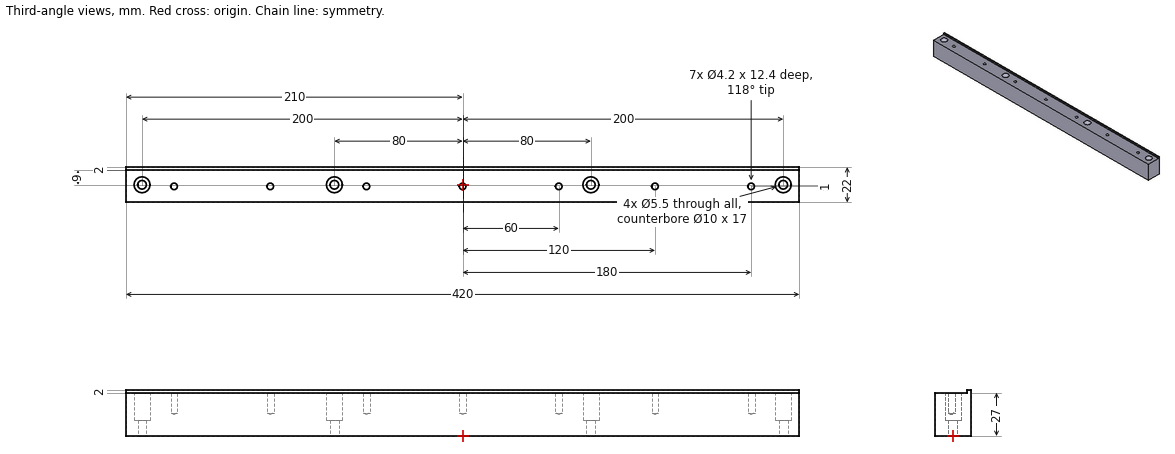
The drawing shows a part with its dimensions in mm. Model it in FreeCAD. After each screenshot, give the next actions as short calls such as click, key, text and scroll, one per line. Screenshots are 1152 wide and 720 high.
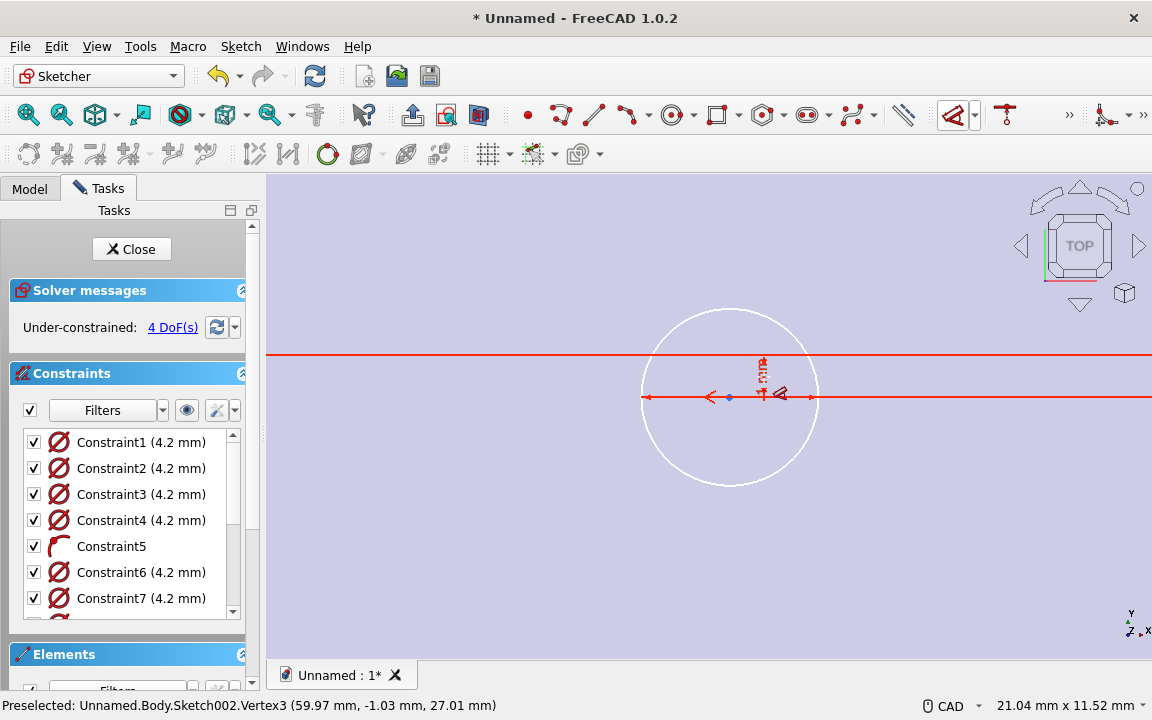
scroll(744, 417, down, 16)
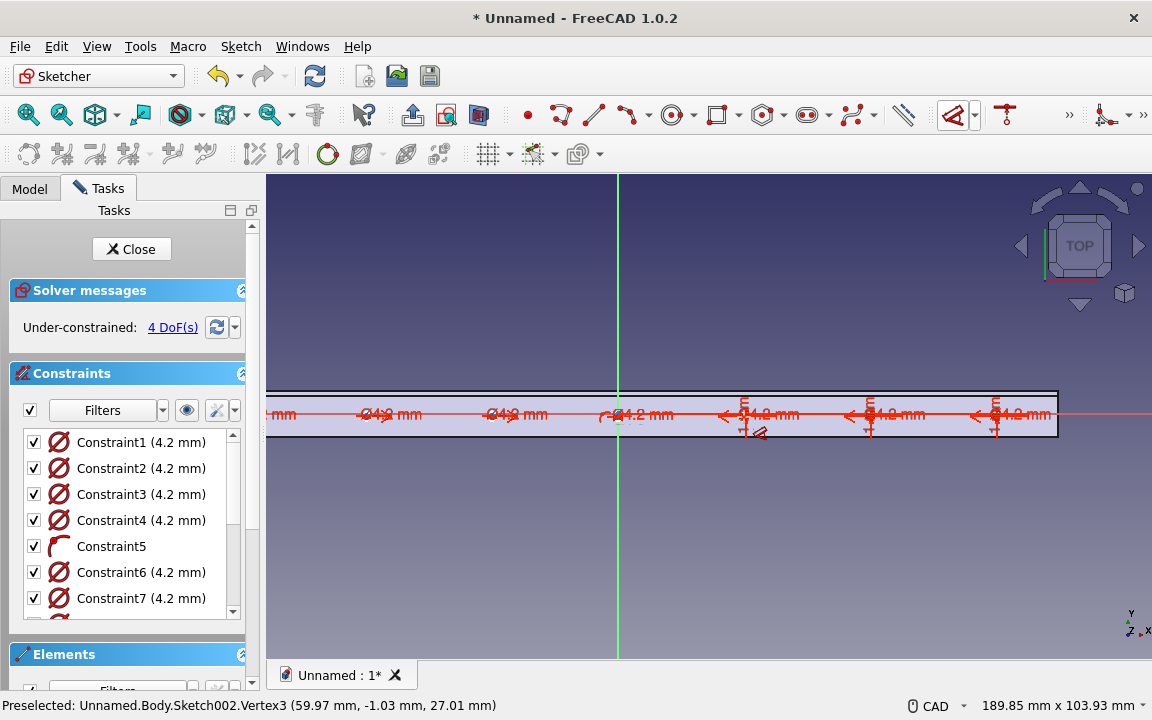
scroll(641, 417, up, 16)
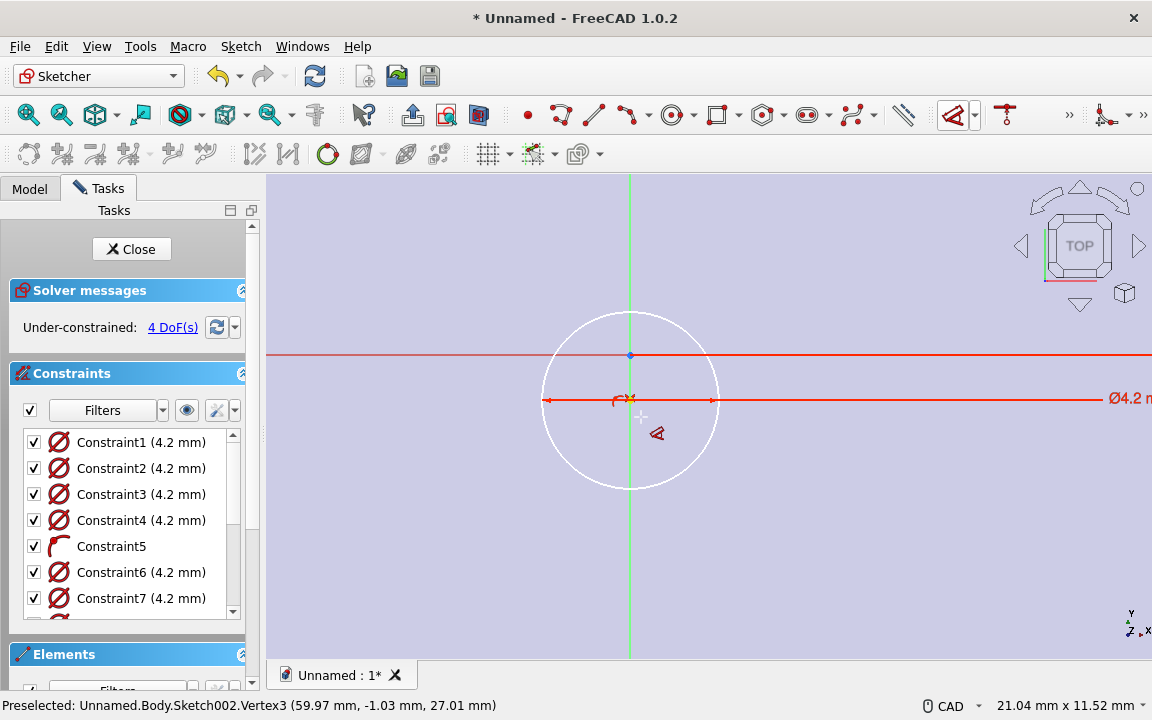
click(630, 400)
click(664, 378)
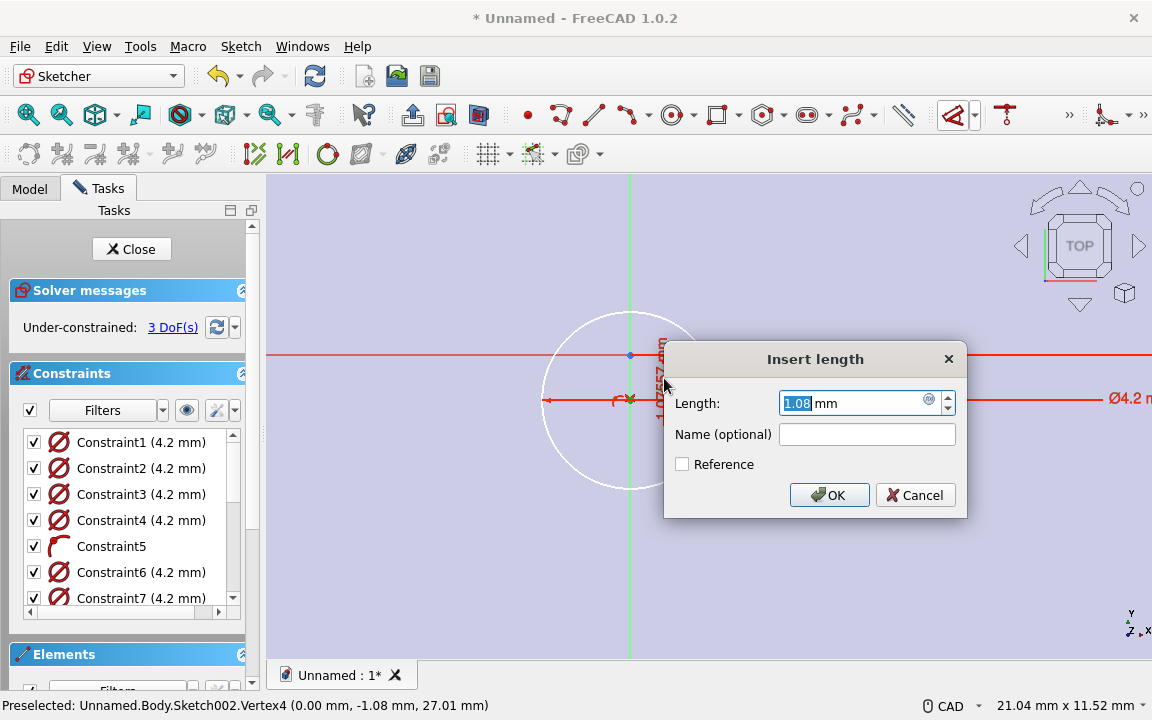
text(1)
key(Return)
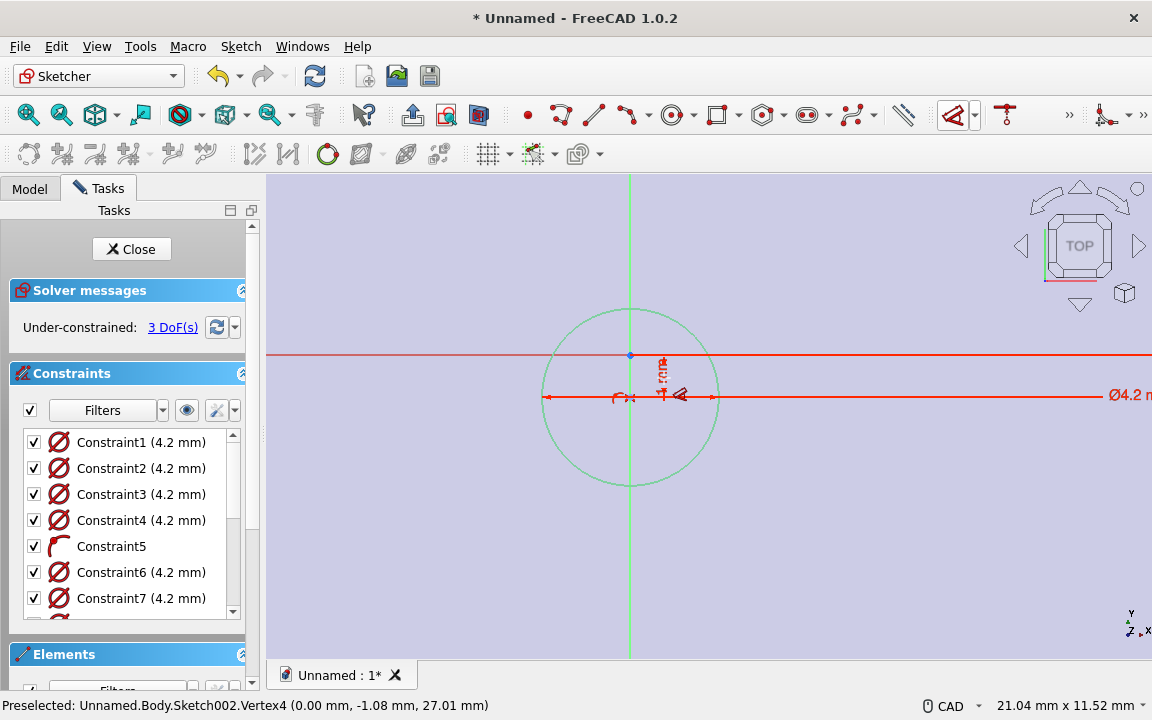
scroll(641, 417, down, 16)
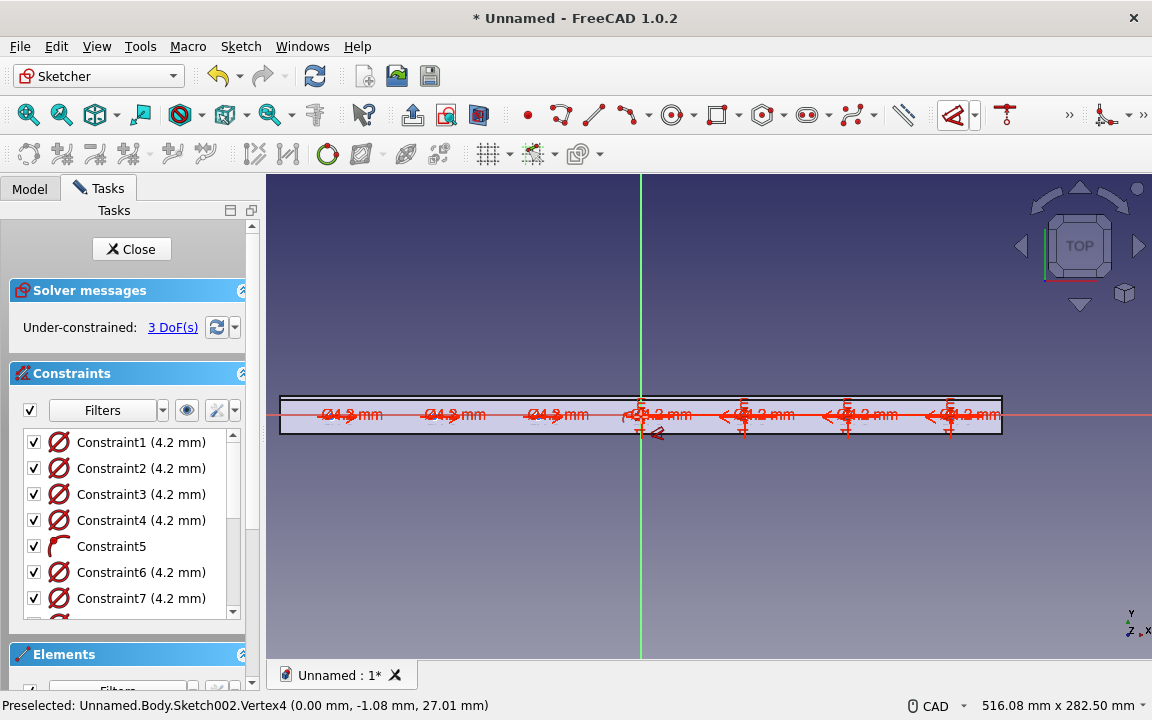
click(744, 417)
click(692, 381)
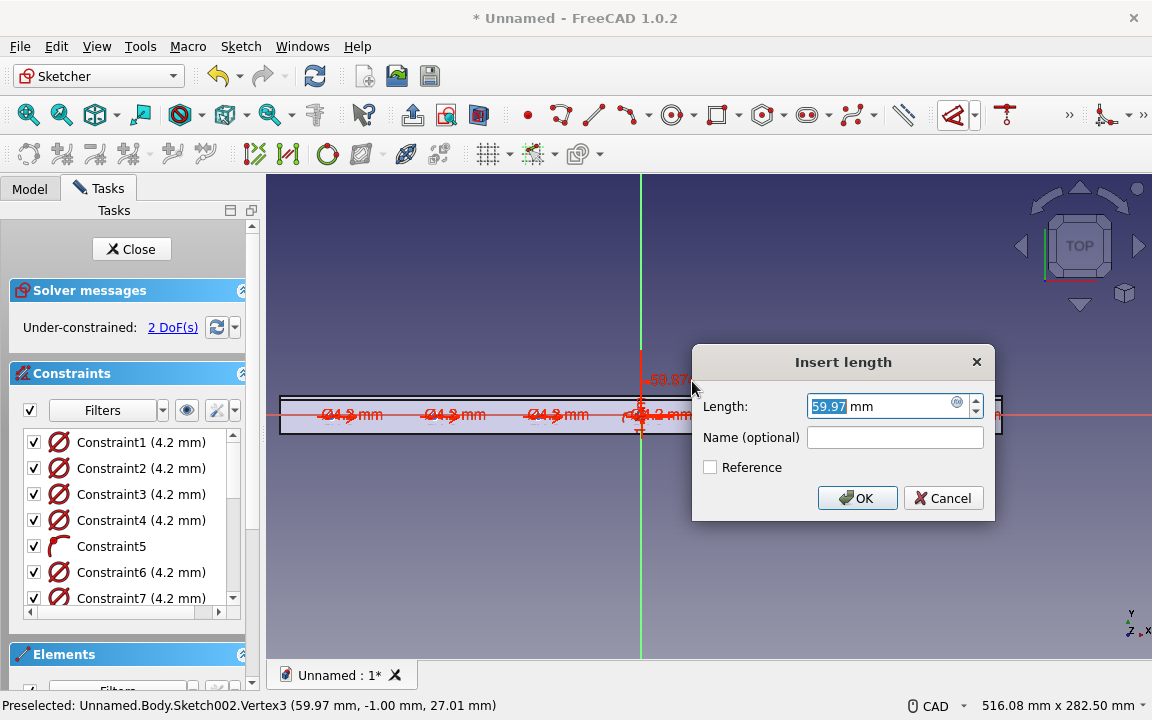
text(60)
key(Return)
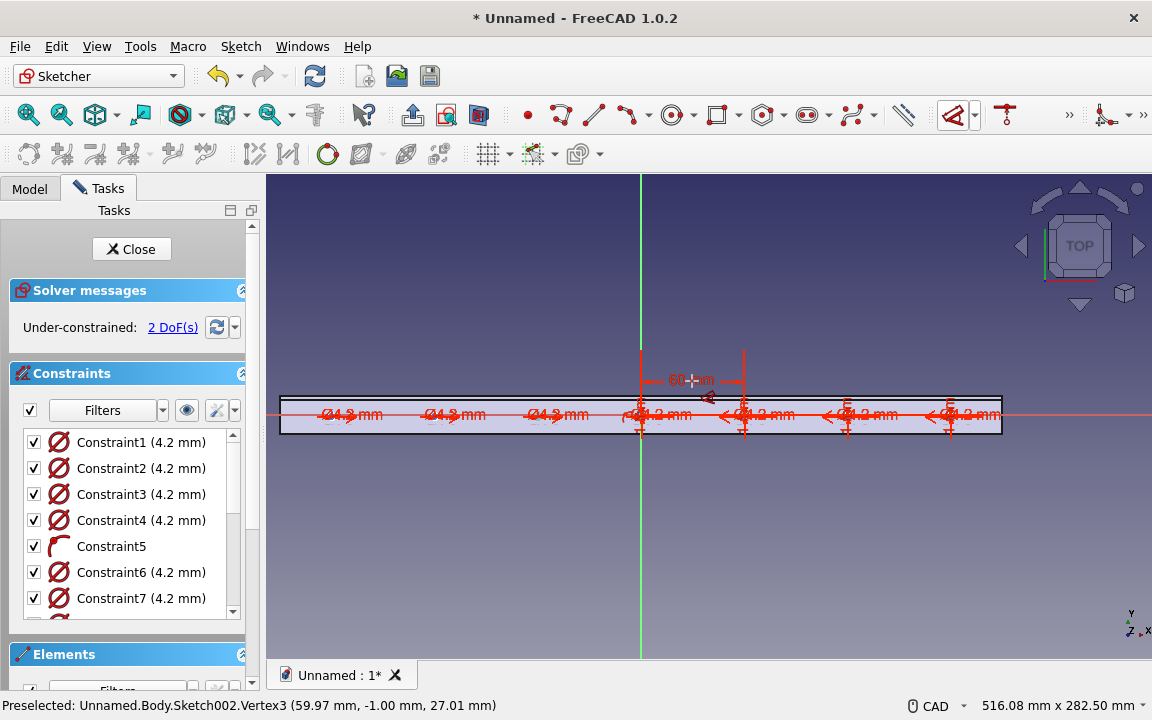
click(950, 417)
click(795, 381)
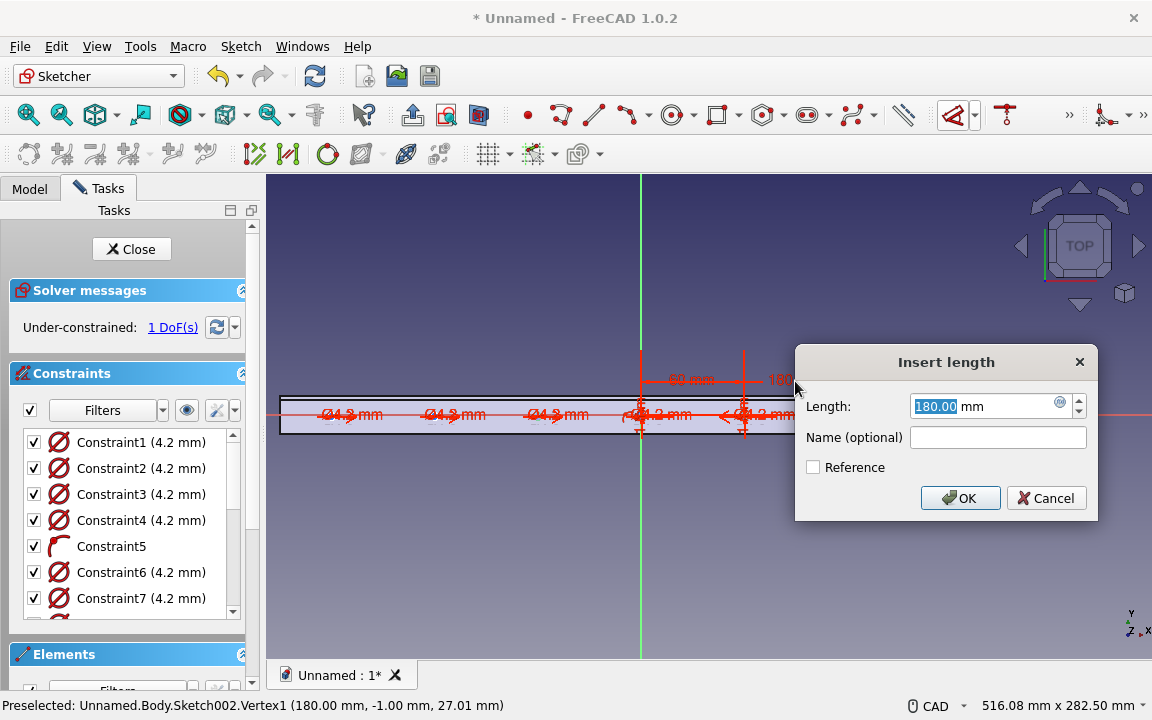
text(180)
key(Return)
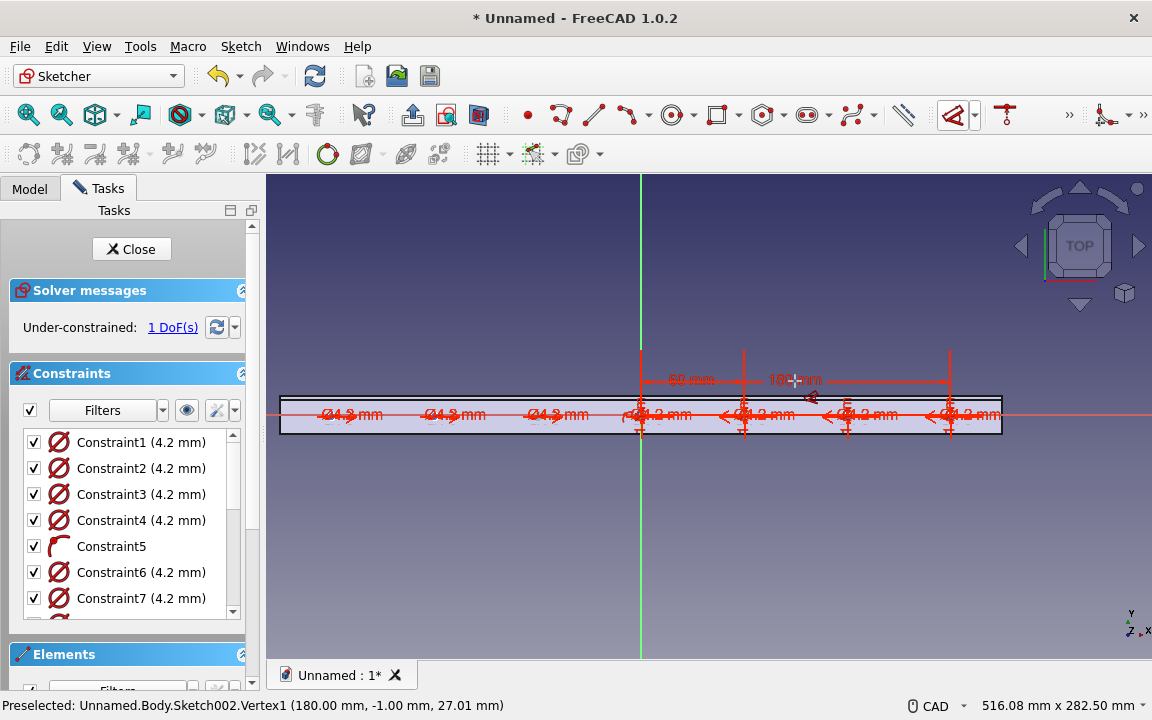
click(847, 417)
click(744, 451)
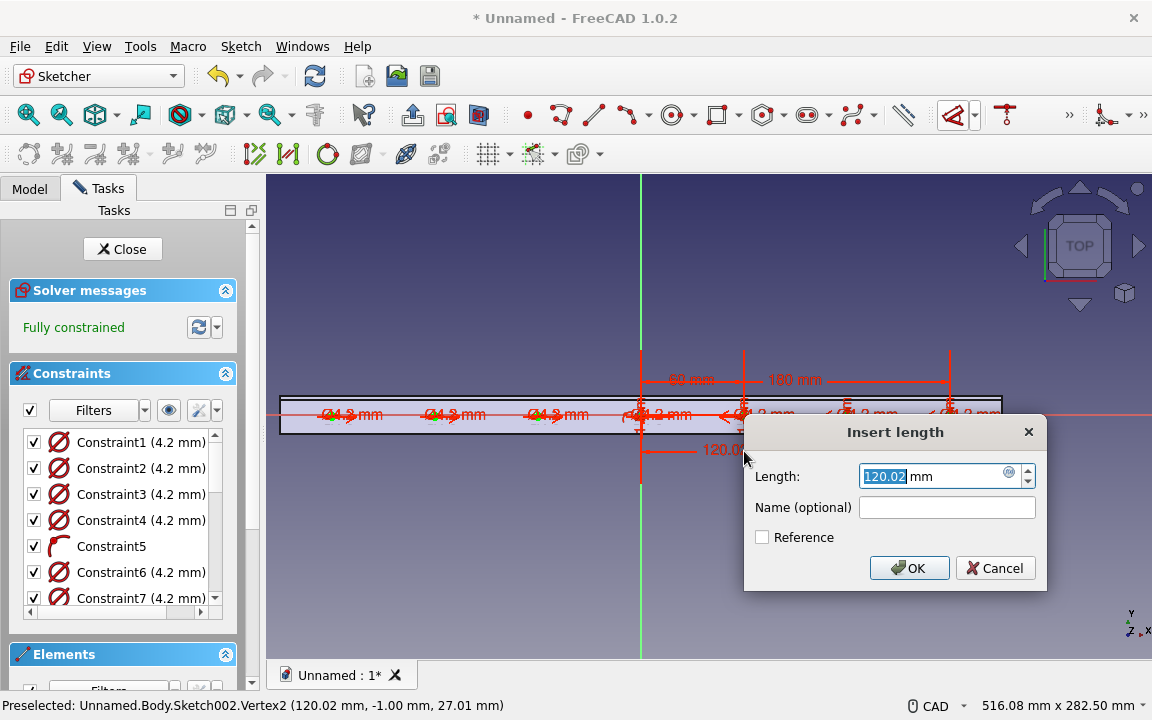
text(120)
key(Return)
key(Escape)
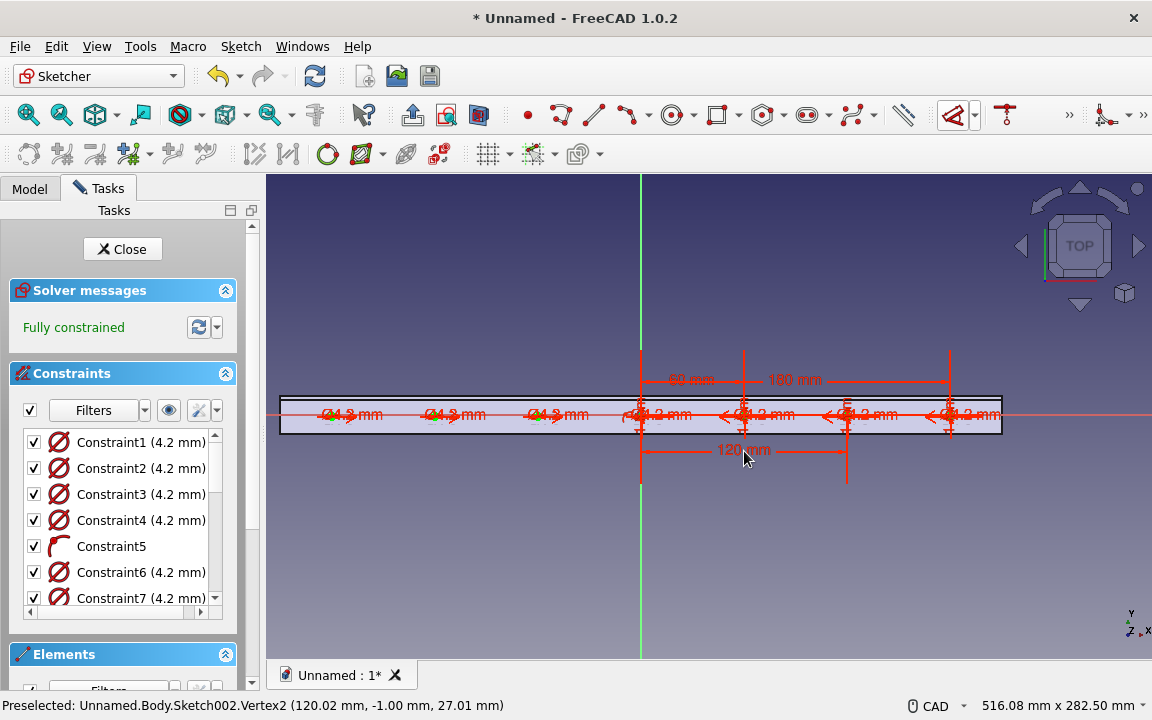
click(123, 249)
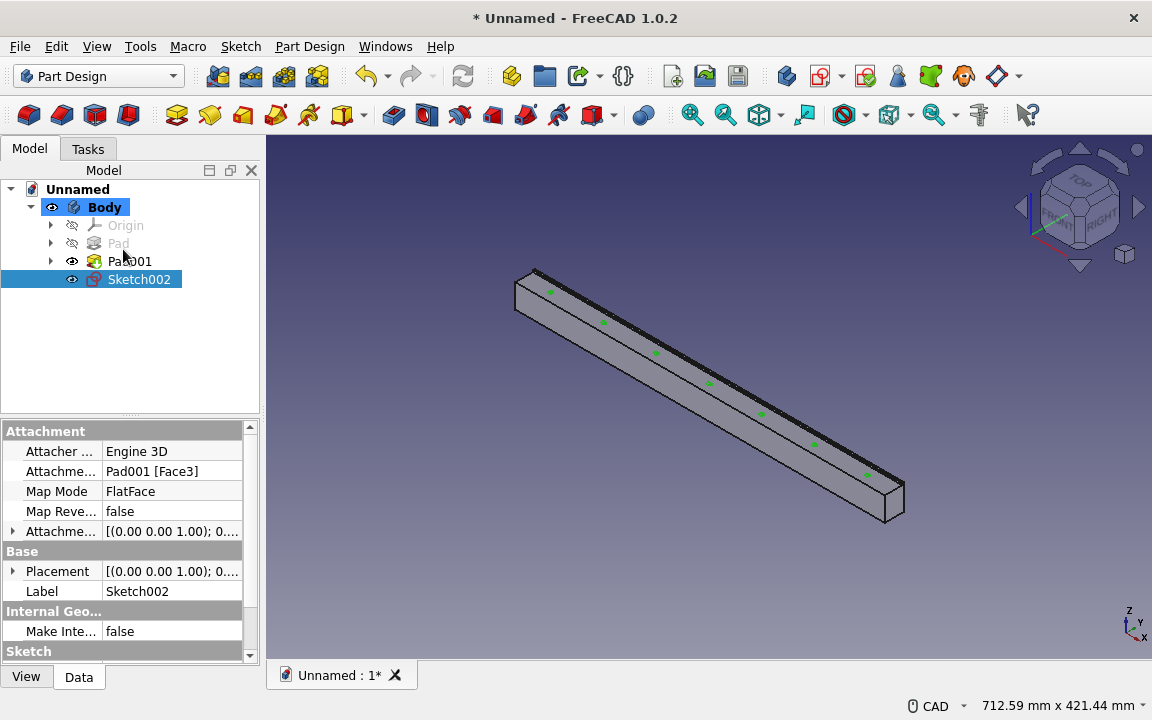
click(427, 116)